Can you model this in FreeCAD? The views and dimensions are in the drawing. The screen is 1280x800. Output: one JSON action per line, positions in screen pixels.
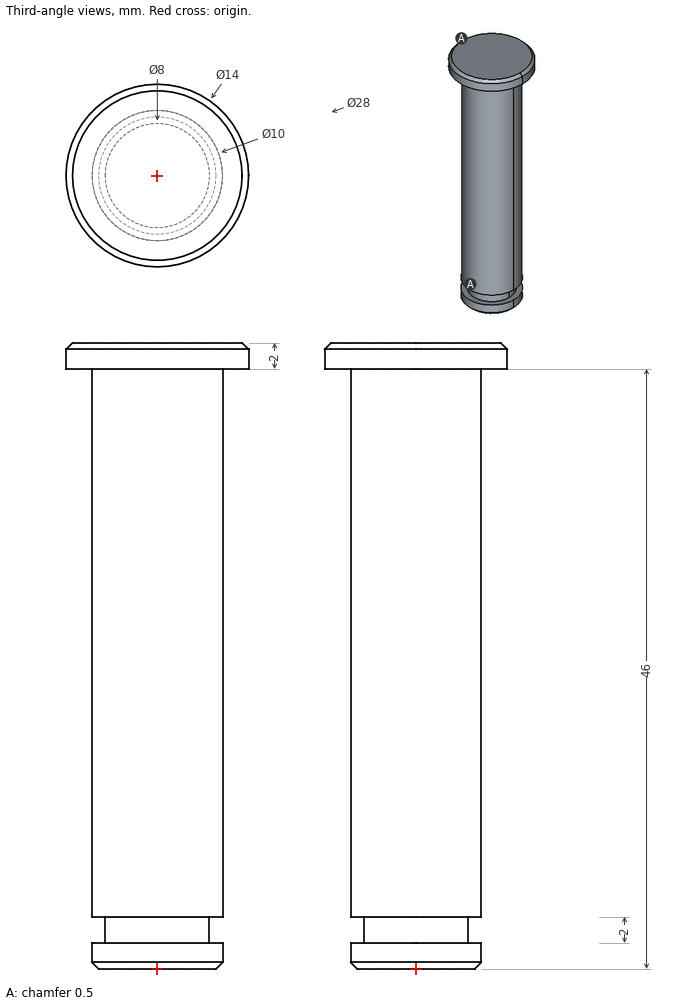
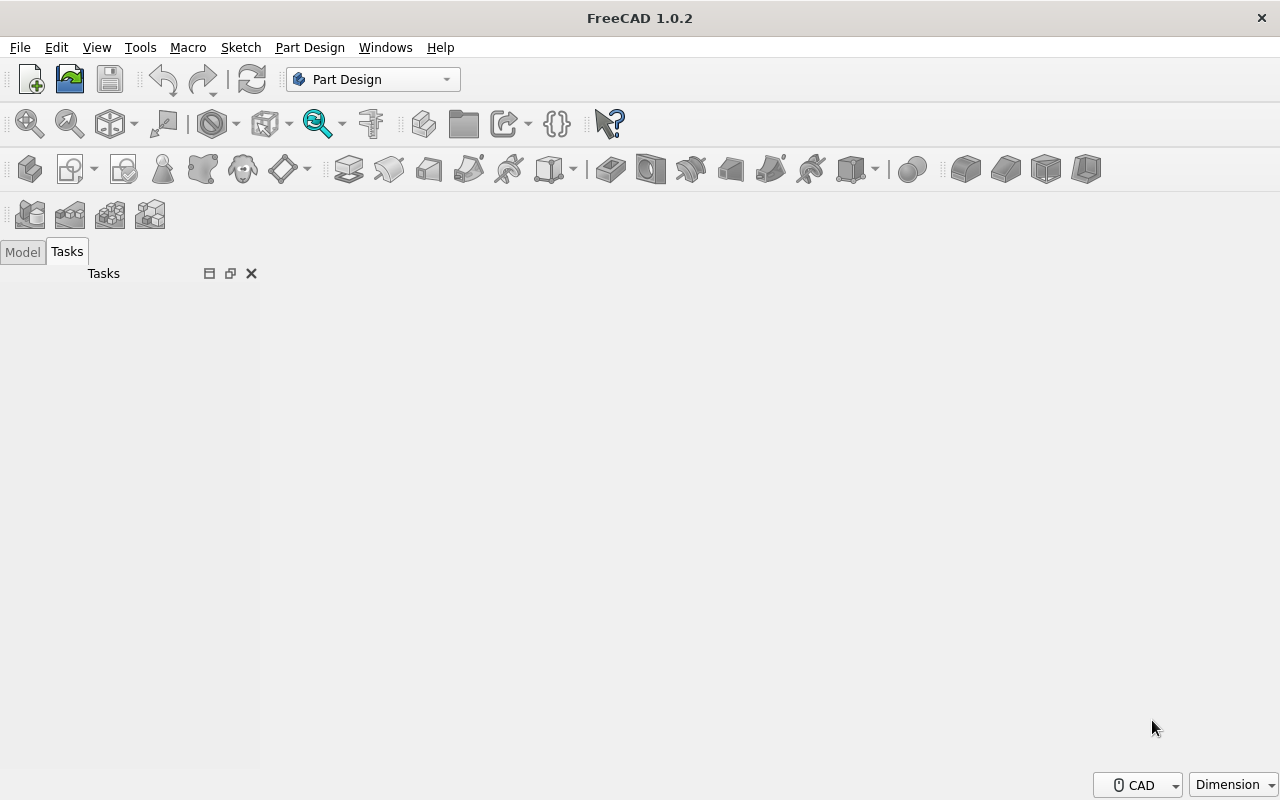
{"action": "key", "text": "ctrl+n"}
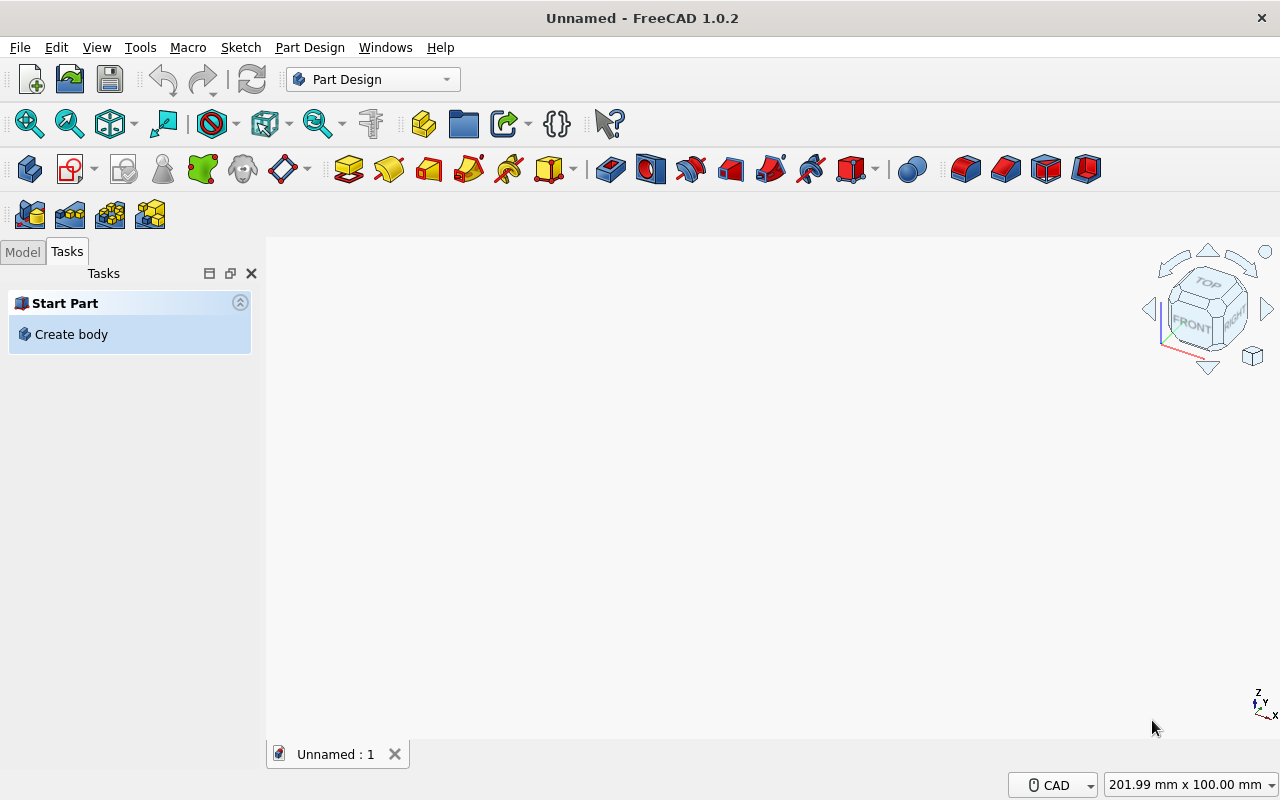
{"action": "left_click", "coordinate": [70, 170]}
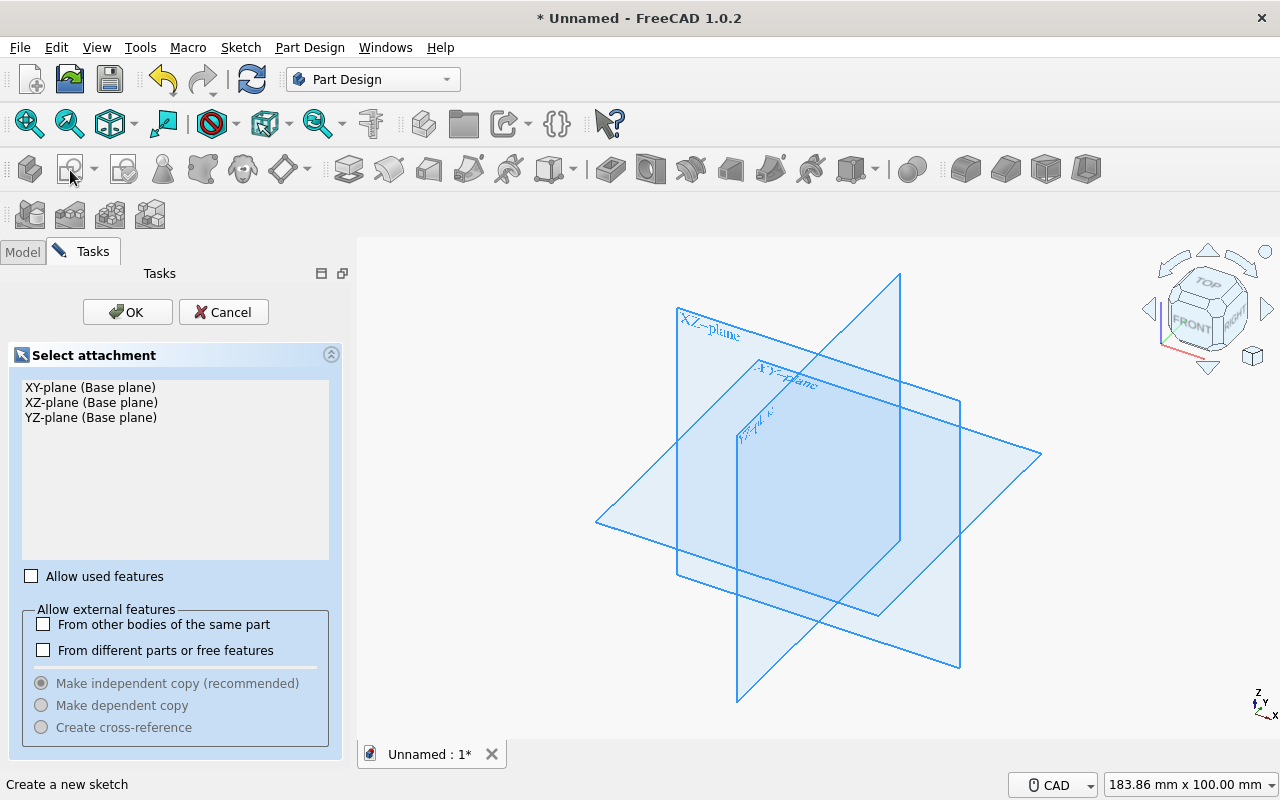
{"action": "left_click", "coordinate": [82, 388]}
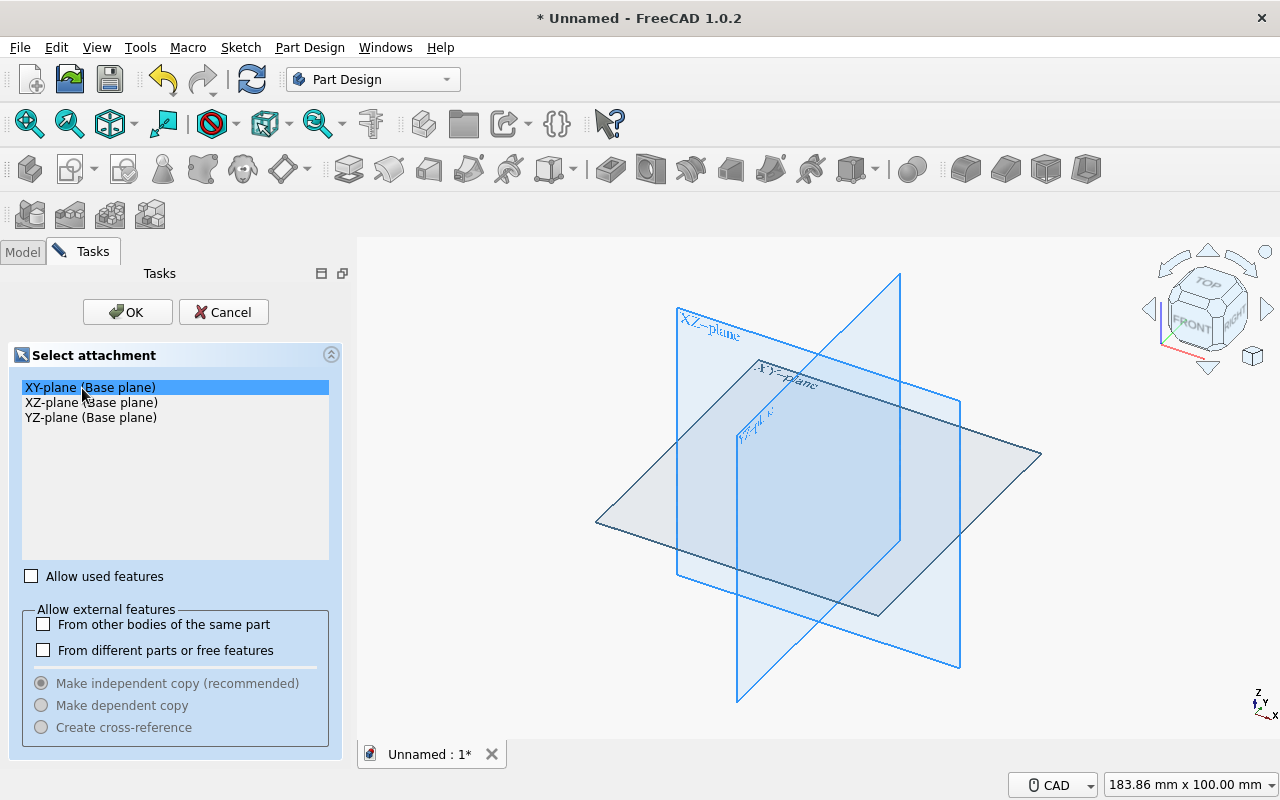
{"action": "left_click", "coordinate": [128, 312]}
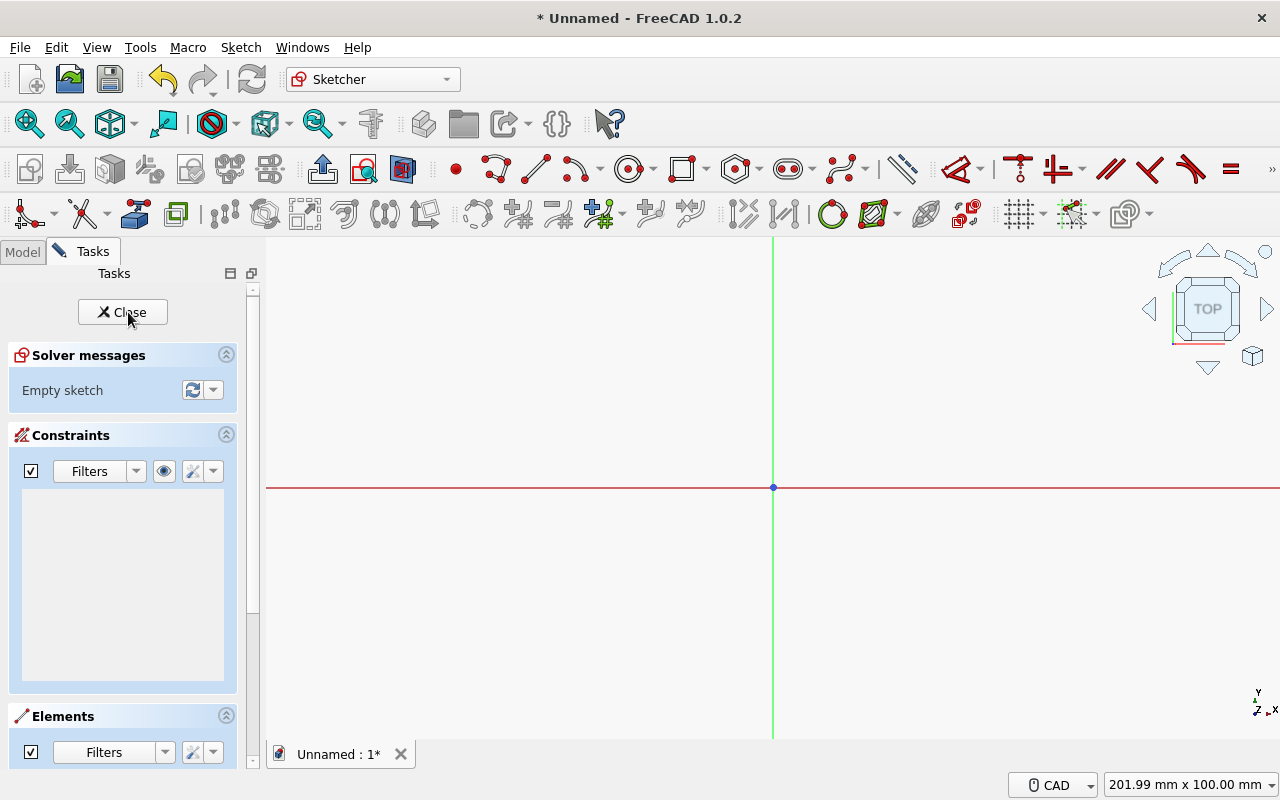
{"action": "scroll", "coordinate": [787, 488], "scroll_direction": "up", "scroll_amount": 9}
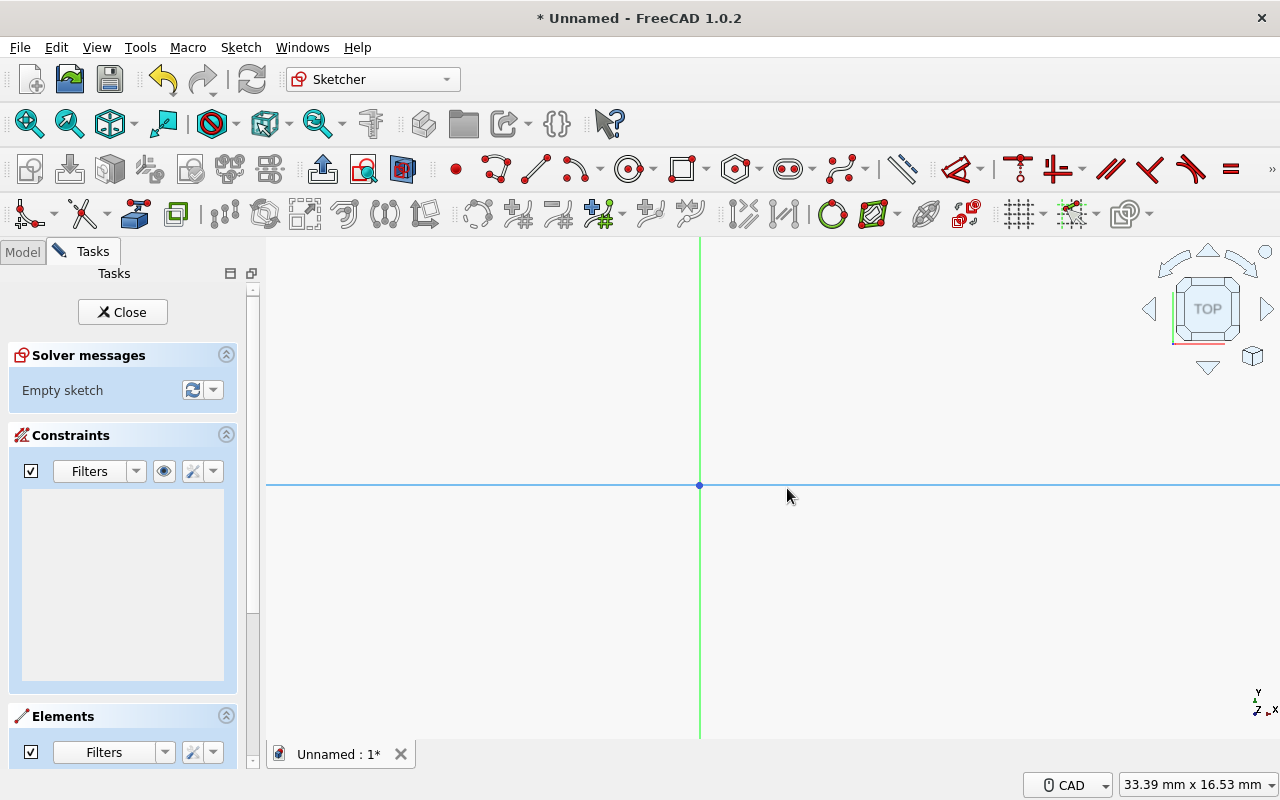
{"action": "left_click", "coordinate": [630, 170]}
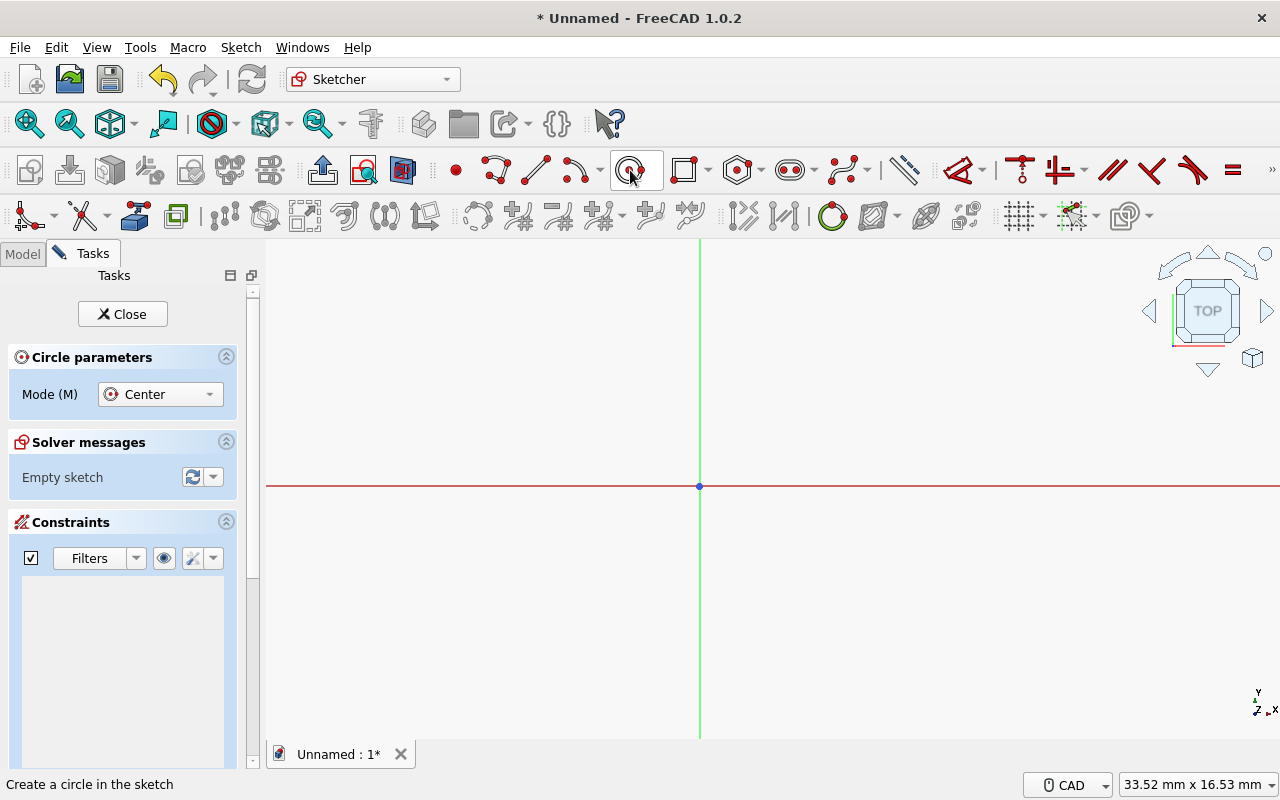
{"action": "left_click", "coordinate": [700, 486]}
{"action": "mouse_move", "coordinate": [807, 380]}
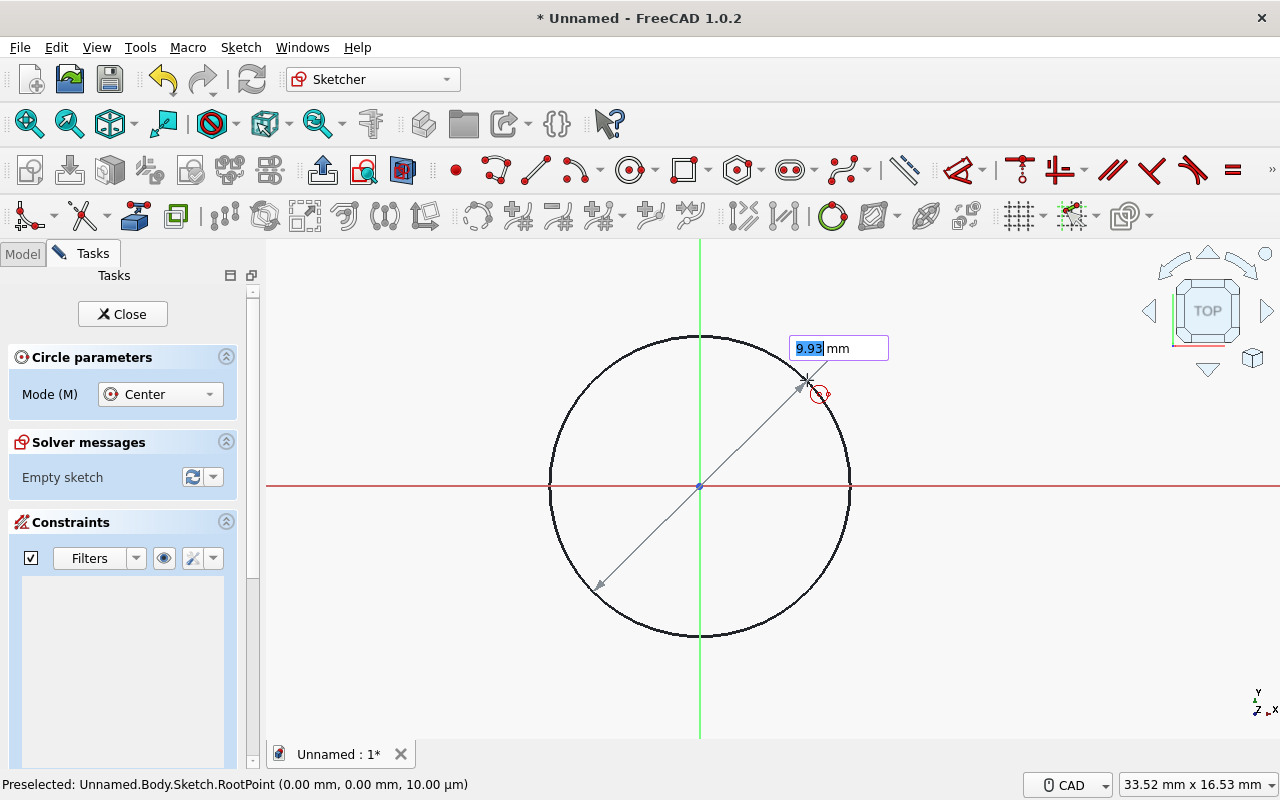
{"action": "type", "text": "10"}
{"action": "key", "text": "Return"}
{"action": "key", "text": "Escape"}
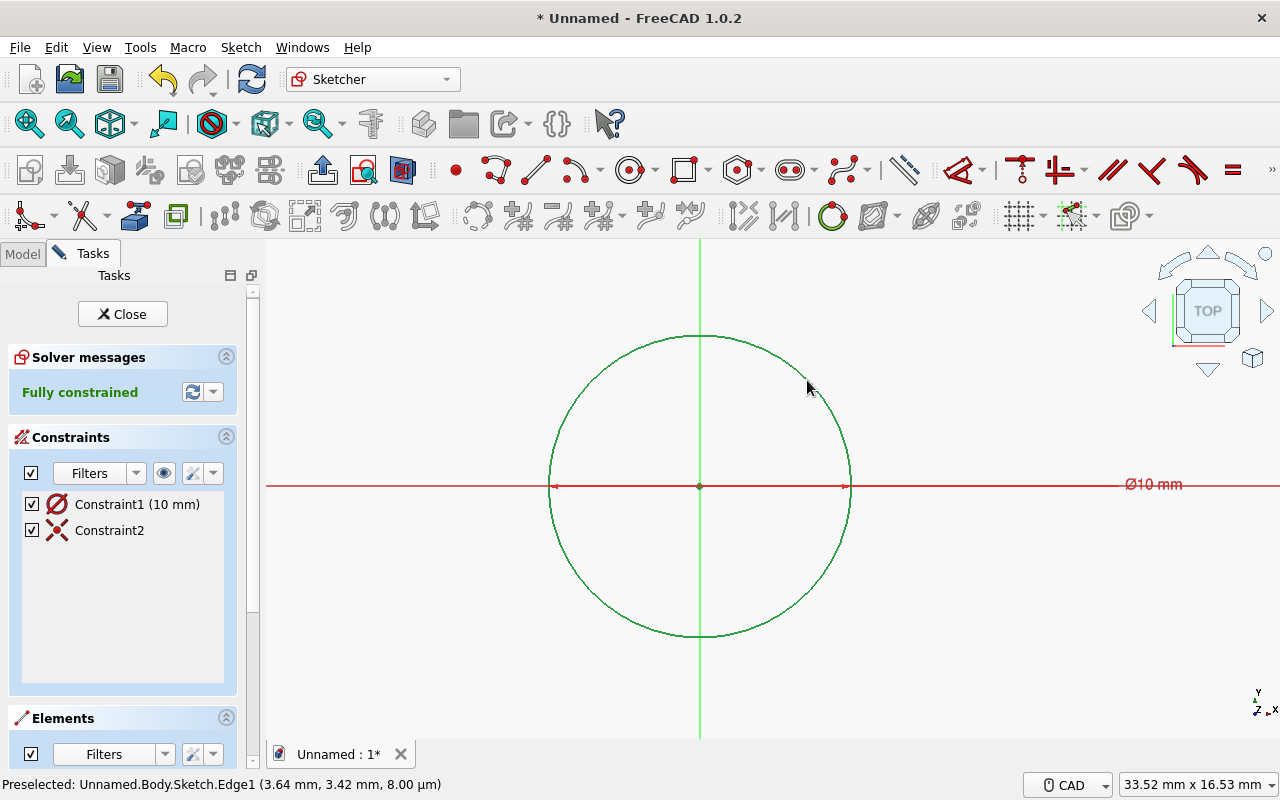
{"action": "left_click", "coordinate": [123, 314]}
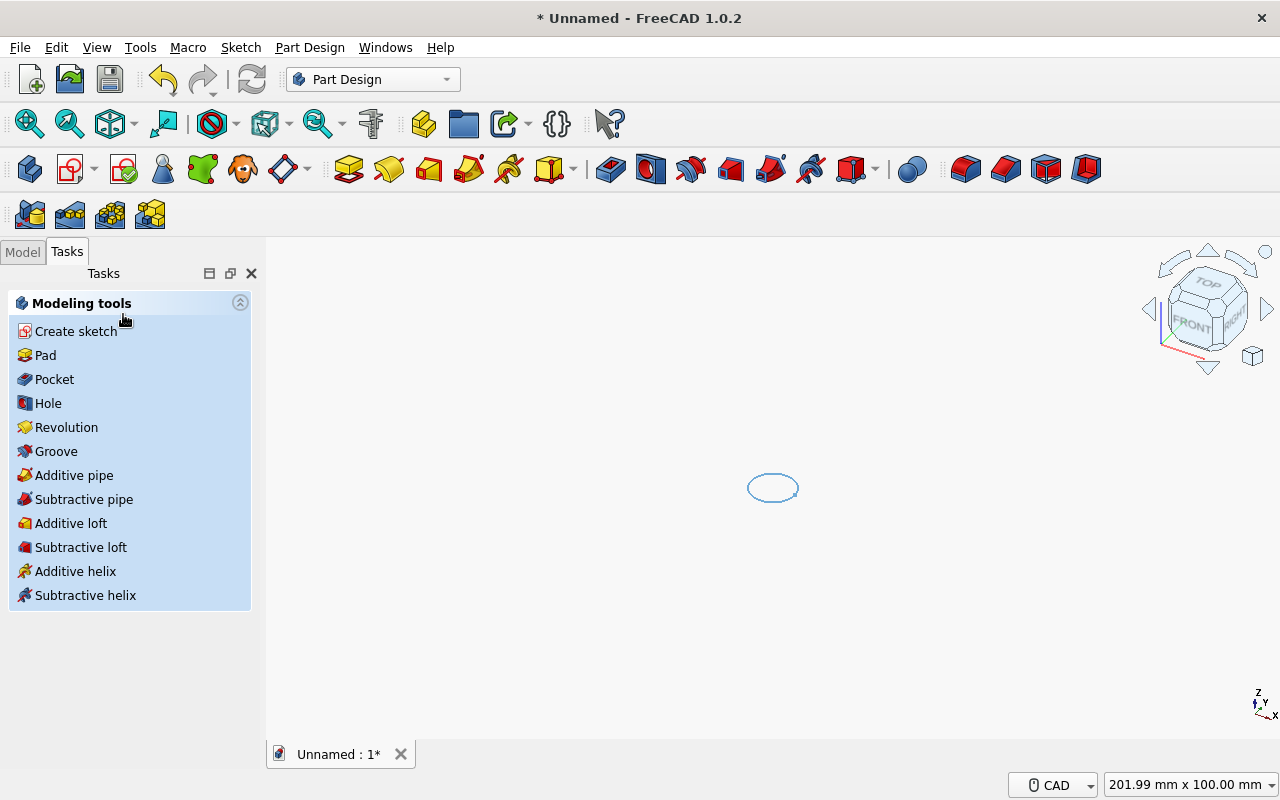
{"action": "left_click", "coordinate": [350, 170]}